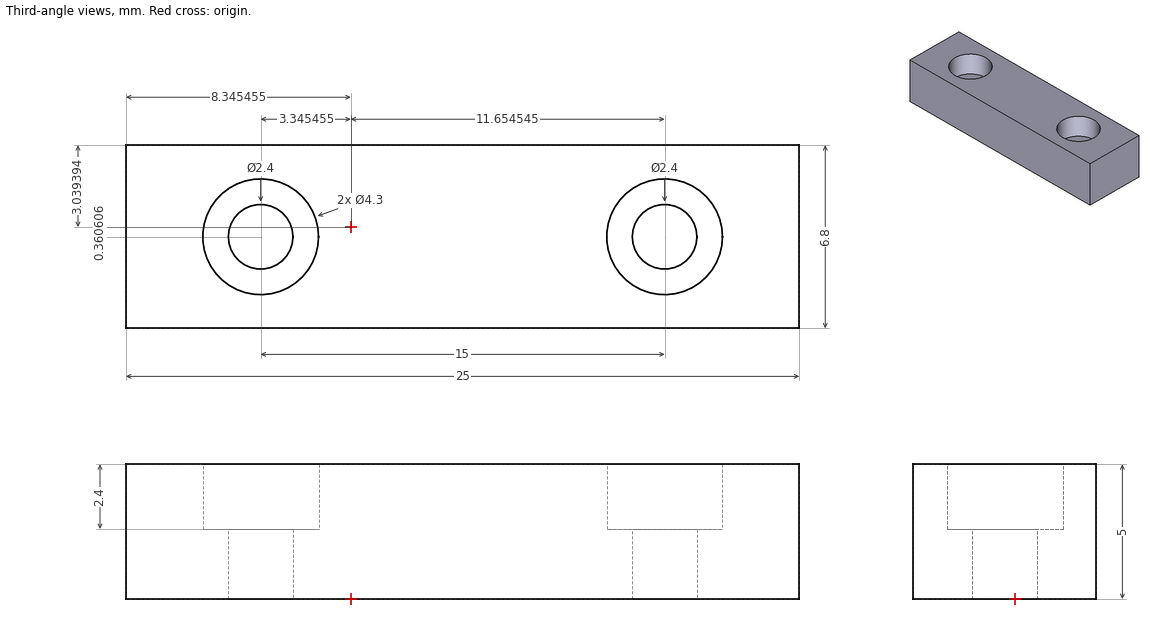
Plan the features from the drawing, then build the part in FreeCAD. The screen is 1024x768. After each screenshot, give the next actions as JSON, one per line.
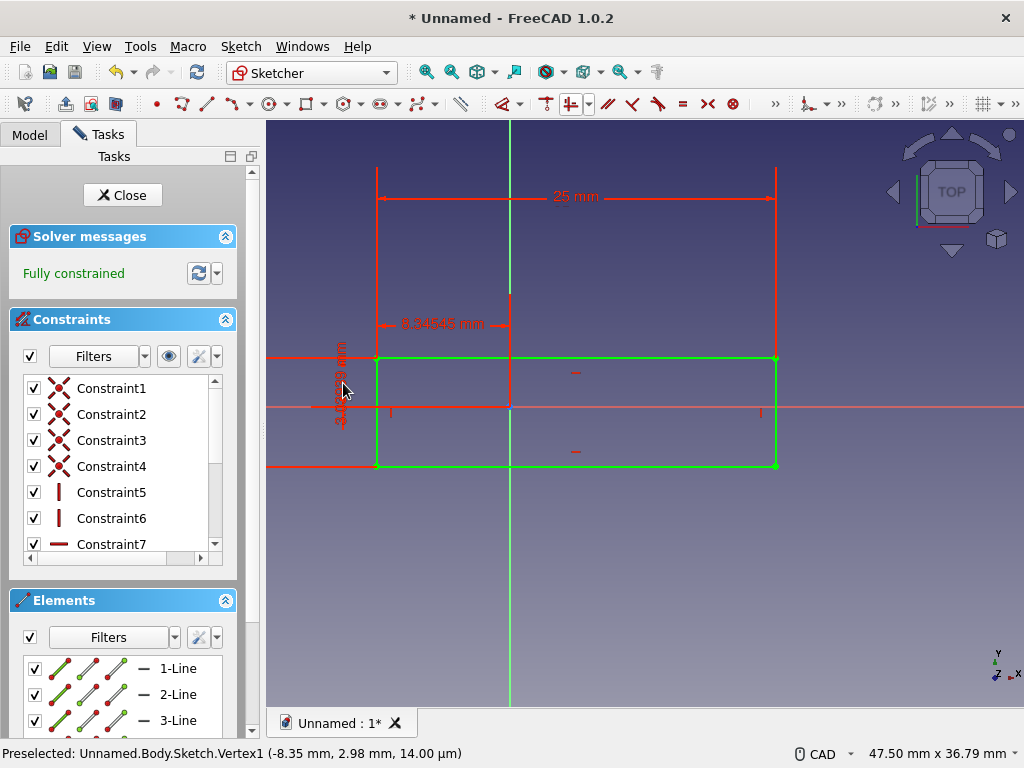
{"action": "left_click", "coordinate": [123, 195]}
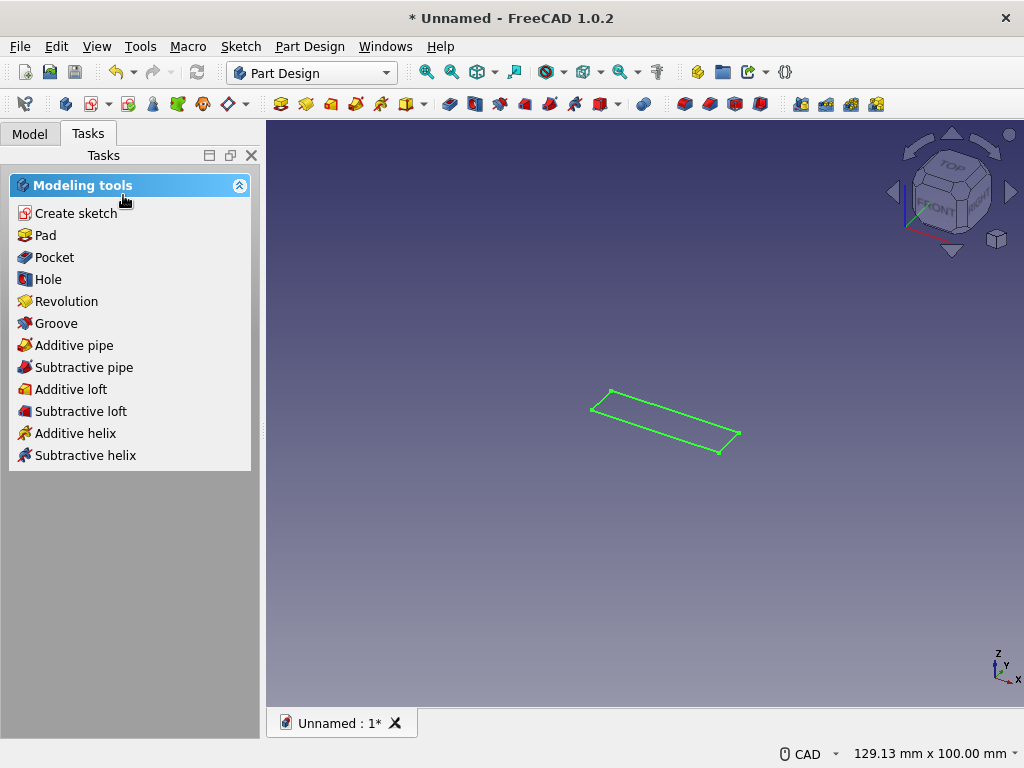
{"action": "left_click", "coordinate": [281, 104]}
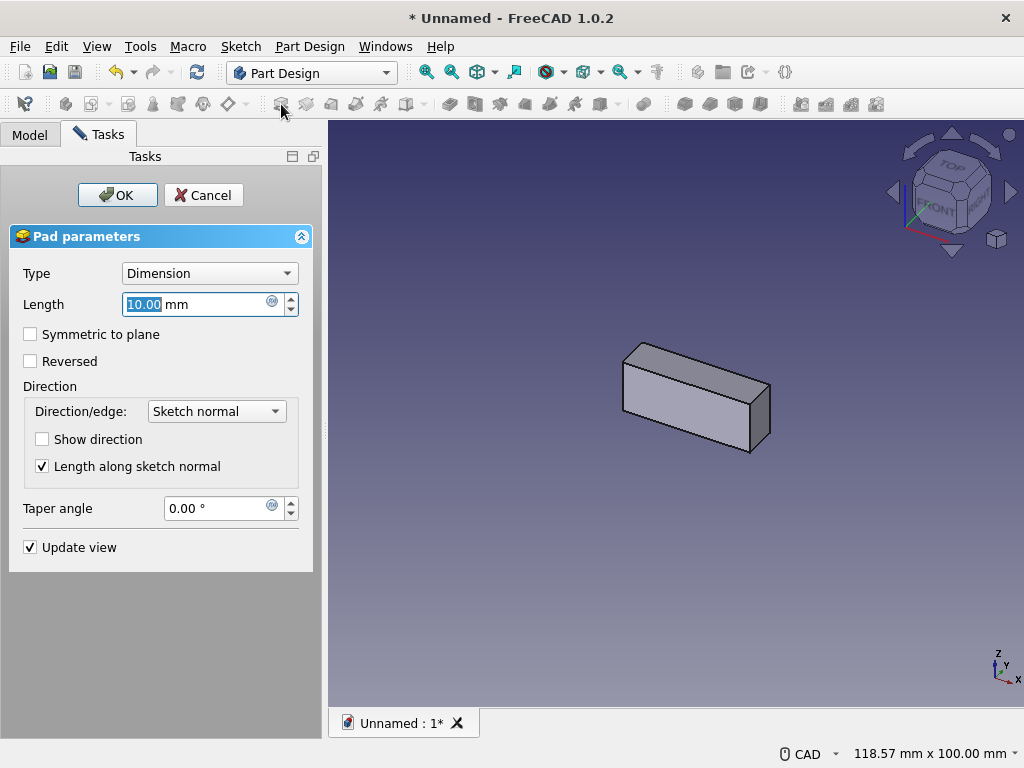
{"action": "type", "text": "5"}
{"action": "key", "text": "Tab"}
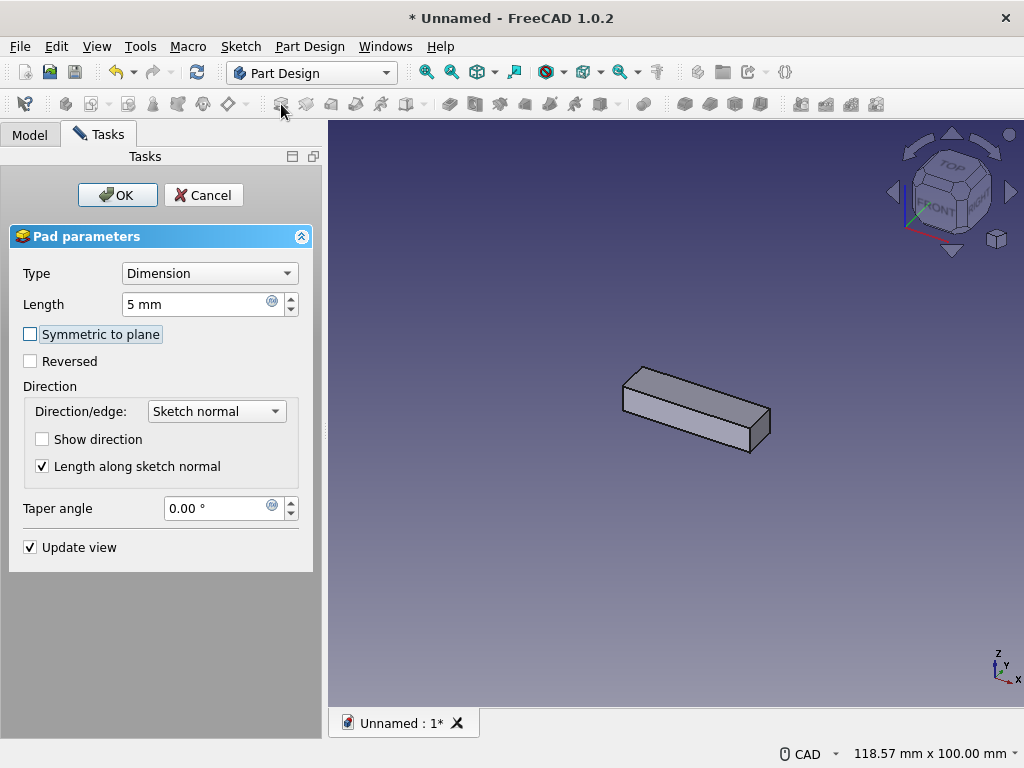
{"action": "left_click", "coordinate": [118, 195]}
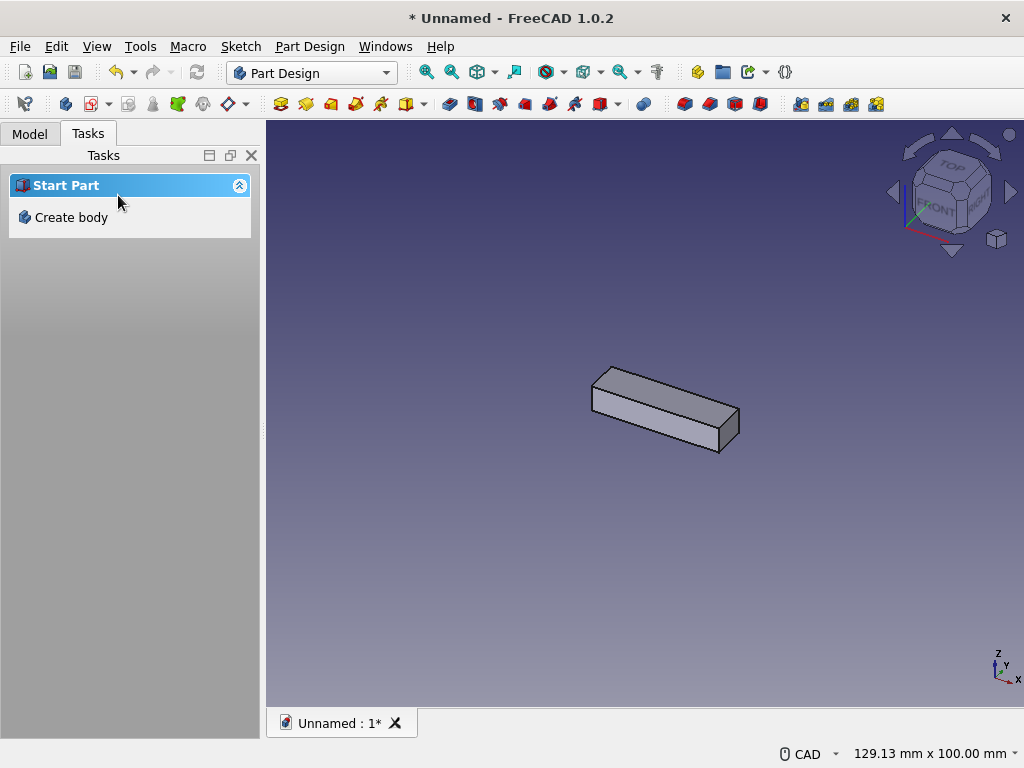
{"action": "left_click", "coordinate": [427, 72]}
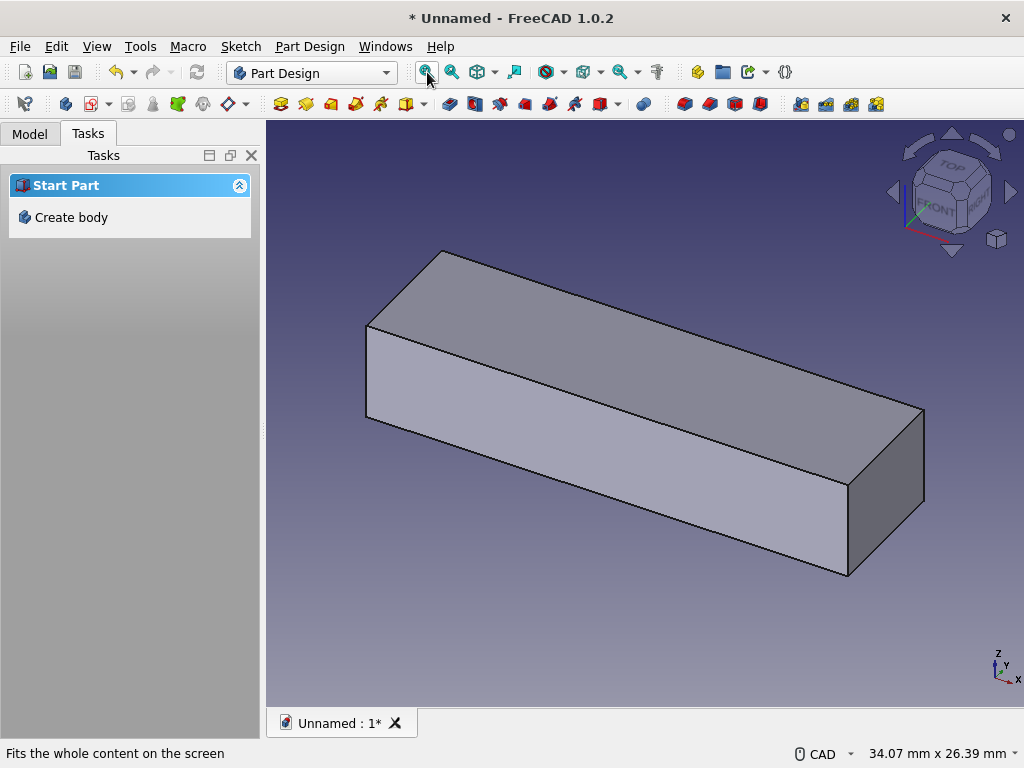
{"action": "left_click", "coordinate": [783, 413]}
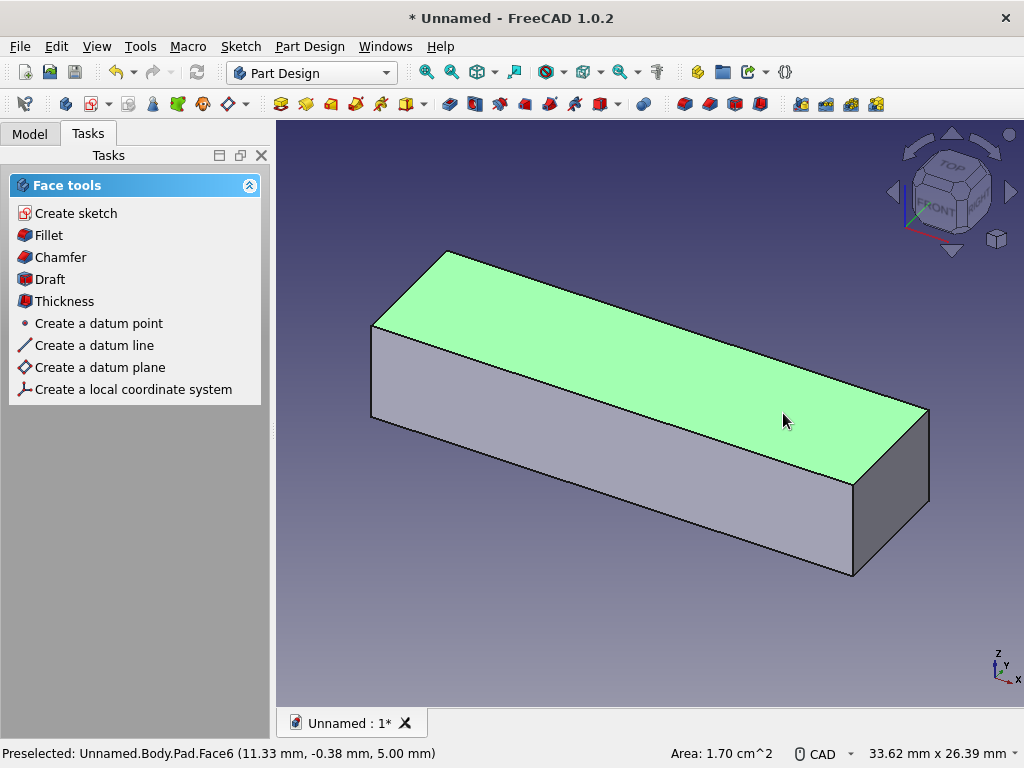
{"action": "left_click", "coordinate": [90, 104]}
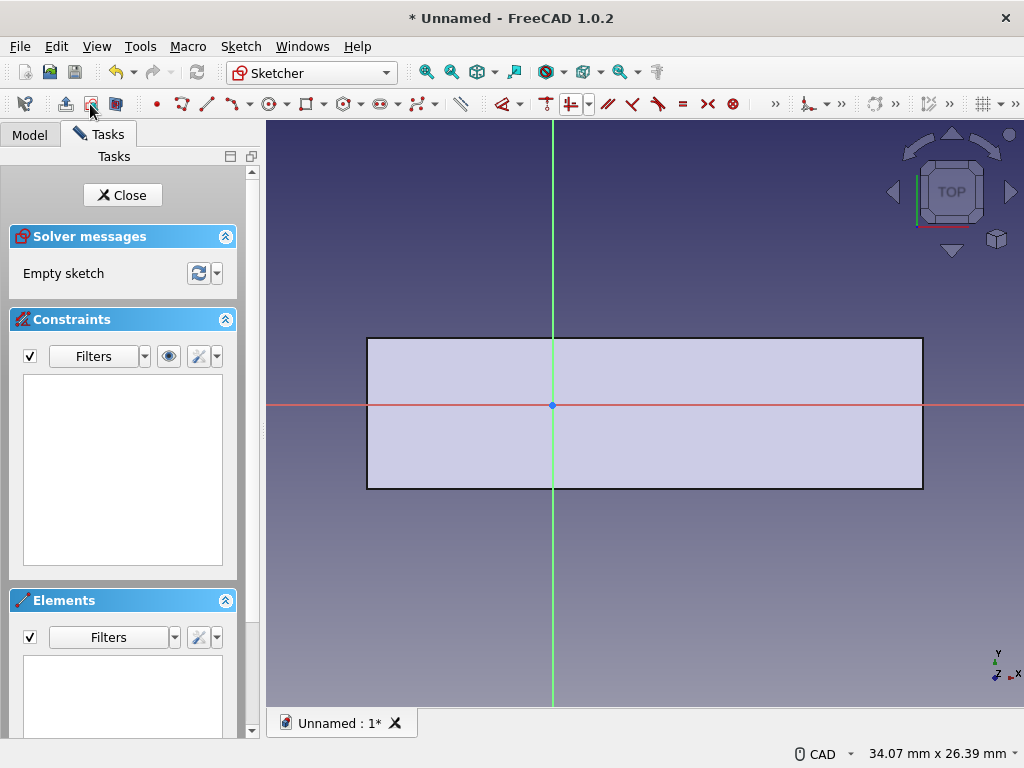
{"action": "scroll", "coordinate": [478, 413], "scroll_direction": "up", "scroll_amount": 7}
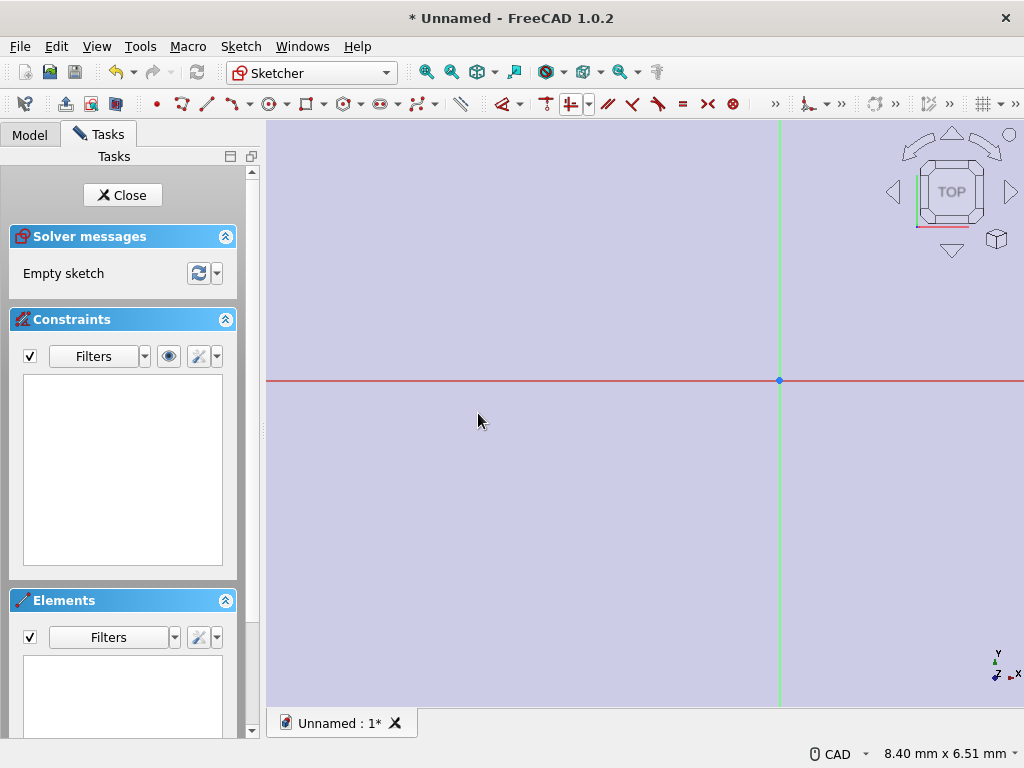
{"action": "left_click", "coordinate": [268, 104]}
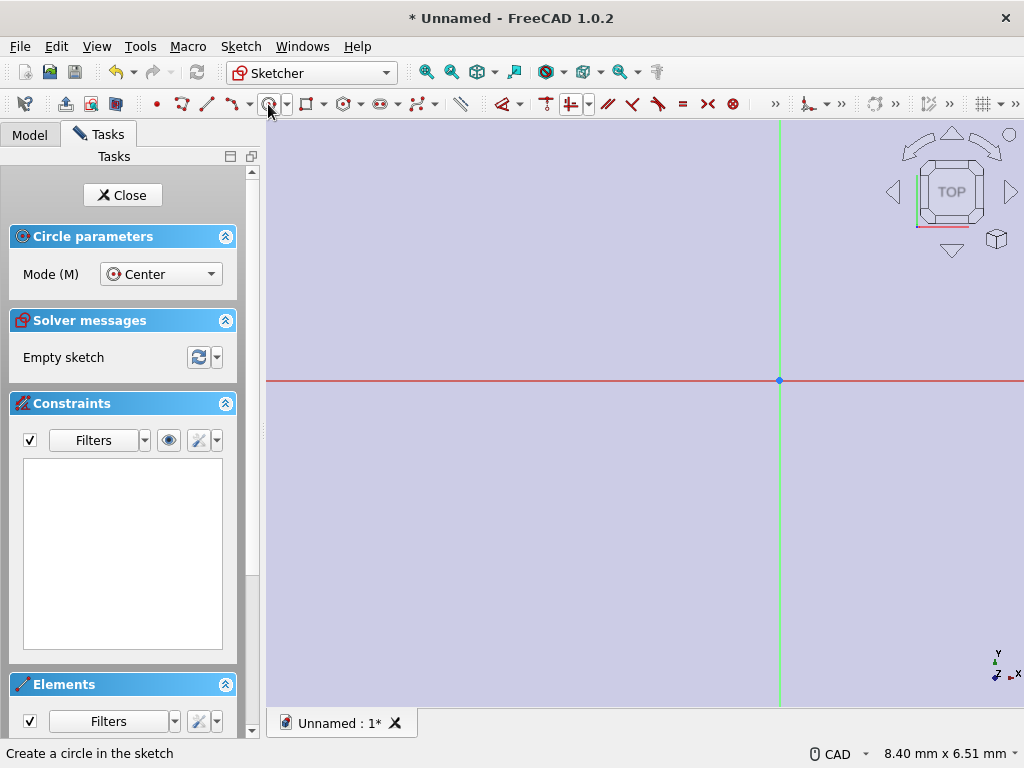
{"action": "left_click", "coordinate": [478, 413]}
{"action": "mouse_move", "coordinate": [554, 337]}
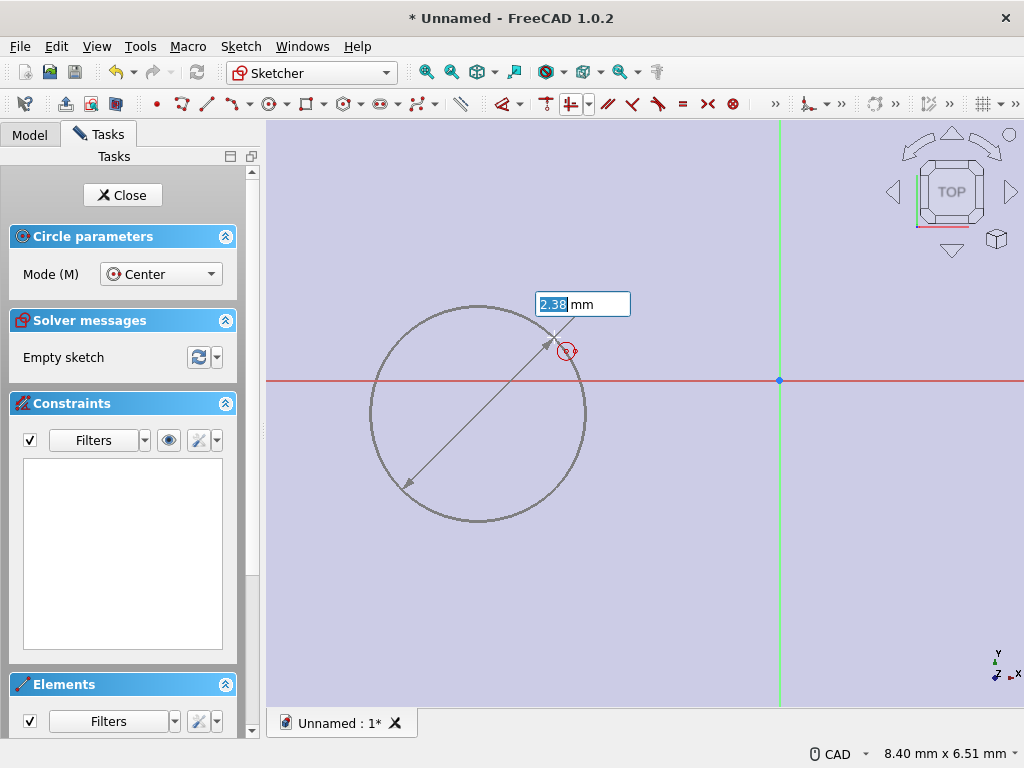
{"action": "type", "text": "2.4"}
{"action": "key", "text": "Return"}
{"action": "key", "text": "Escape"}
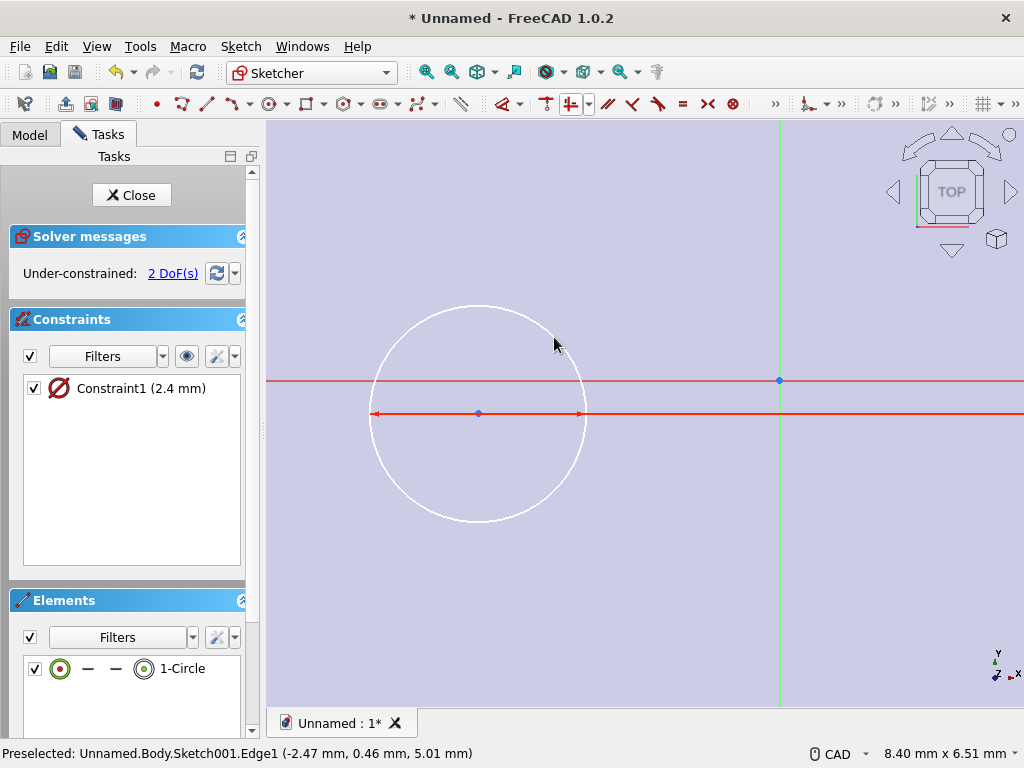
{"action": "left_click", "coordinate": [502, 104]}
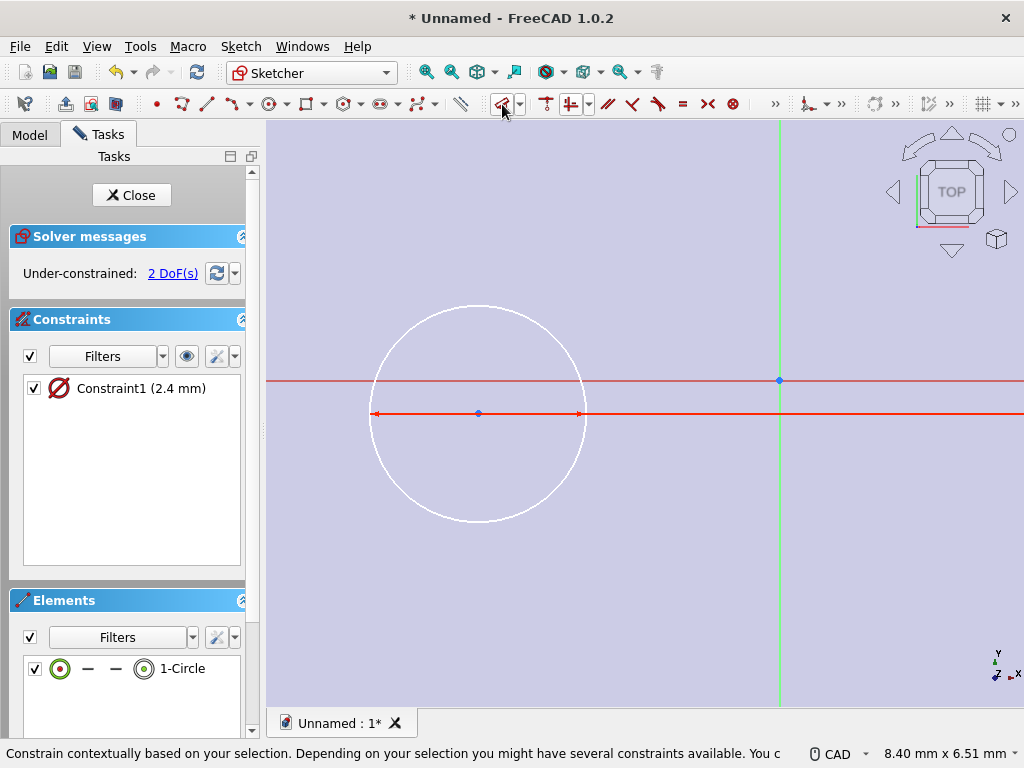
{"action": "left_click", "coordinate": [478, 414]}
{"action": "left_click", "coordinate": [629, 347]}